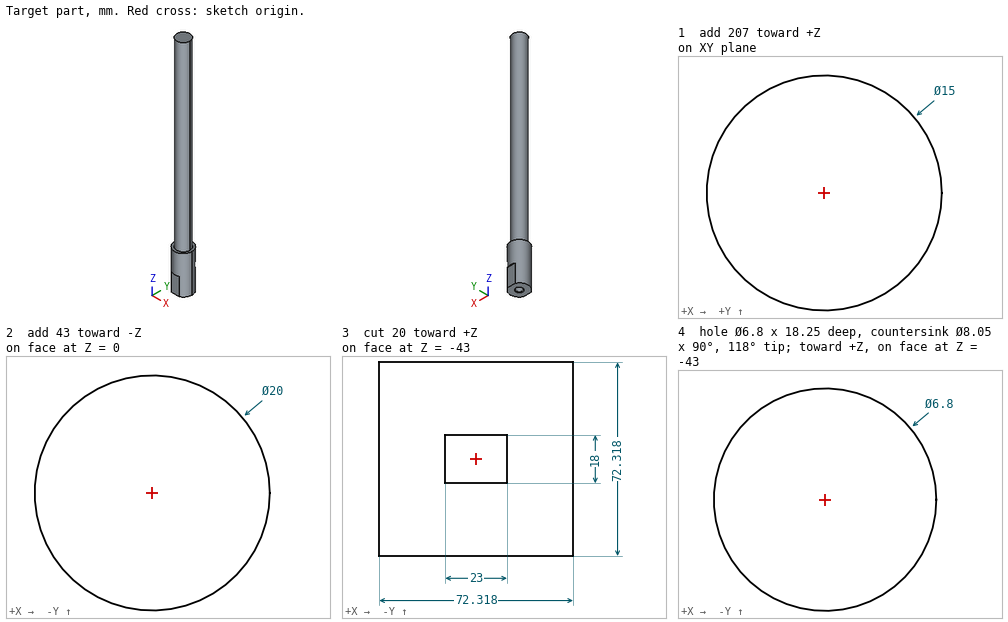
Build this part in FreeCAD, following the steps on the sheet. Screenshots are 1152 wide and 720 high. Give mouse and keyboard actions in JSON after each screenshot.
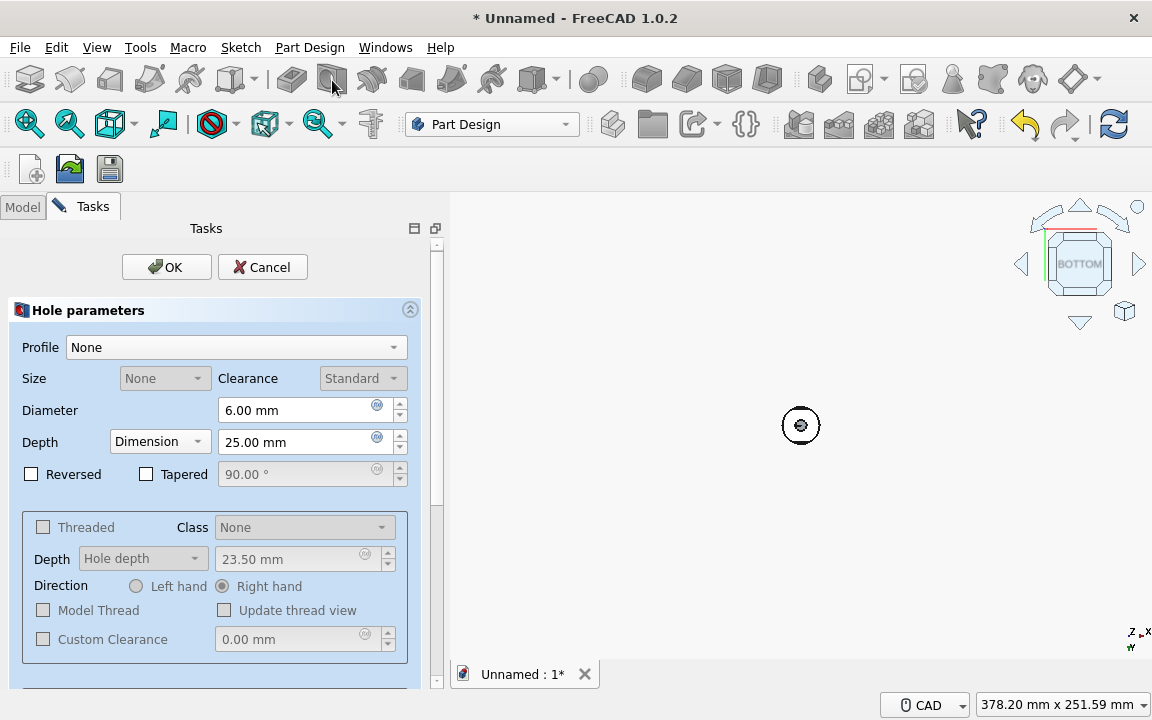
{"action": "triple_click", "coordinate": [305, 410]}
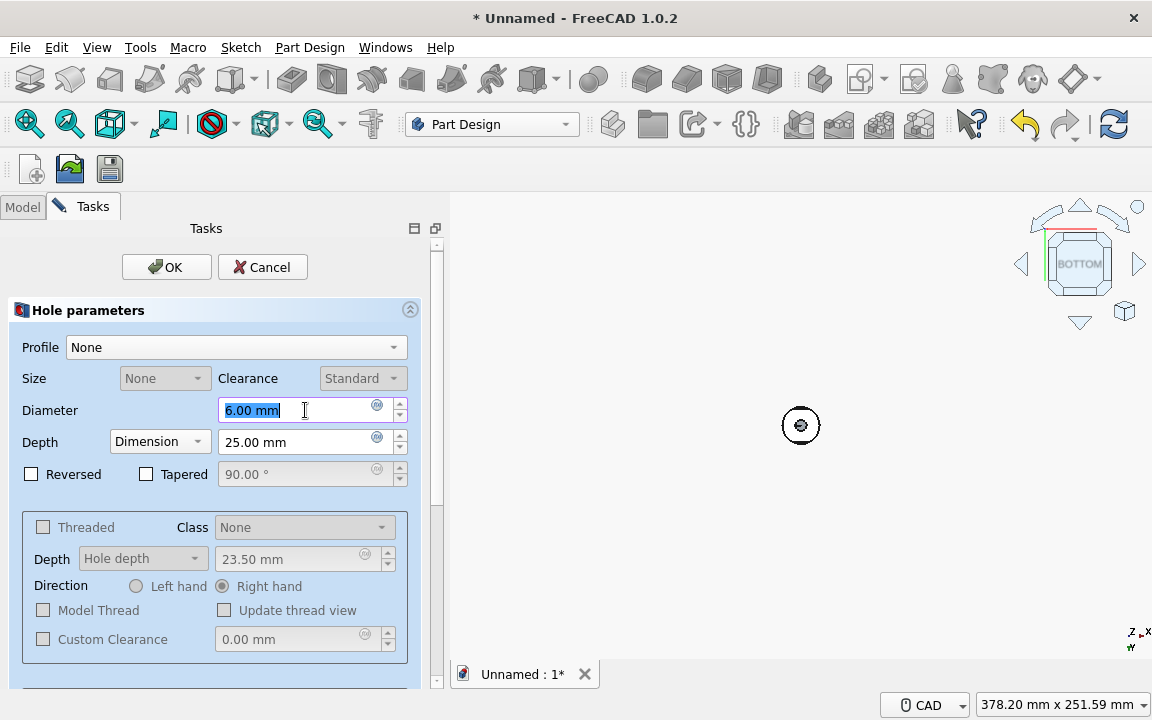
{"action": "type", "text": "6.8"}
{"action": "key", "text": "Tab"}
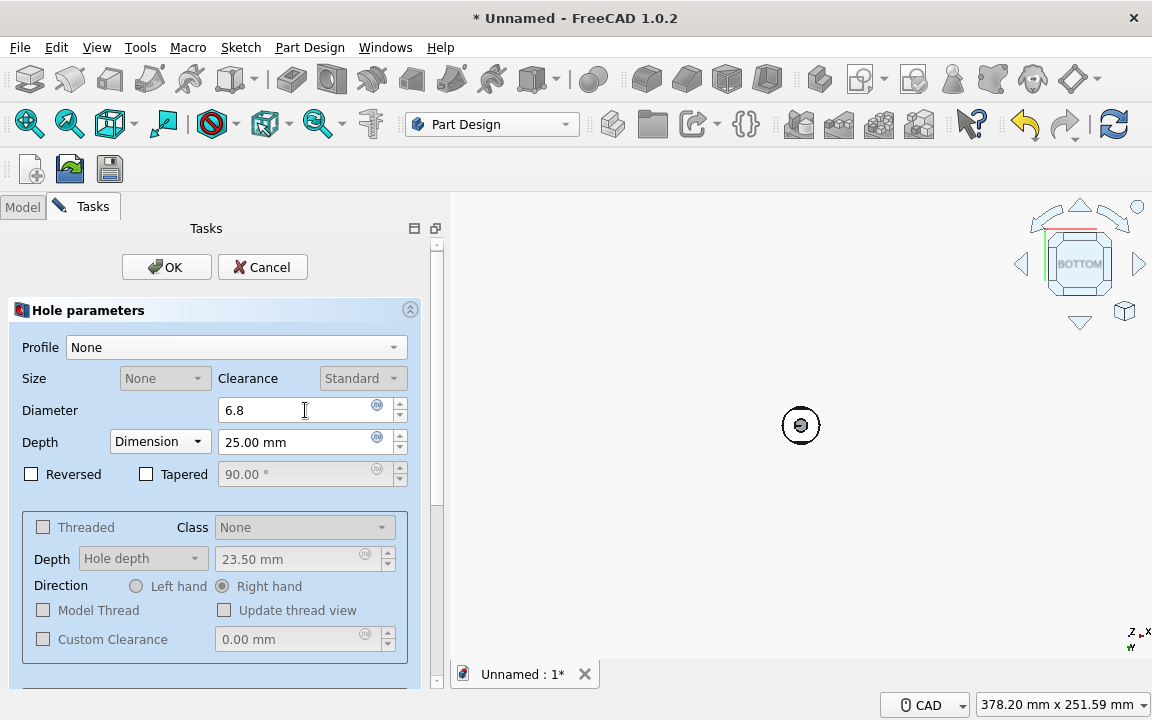
{"action": "triple_click", "coordinate": [305, 442]}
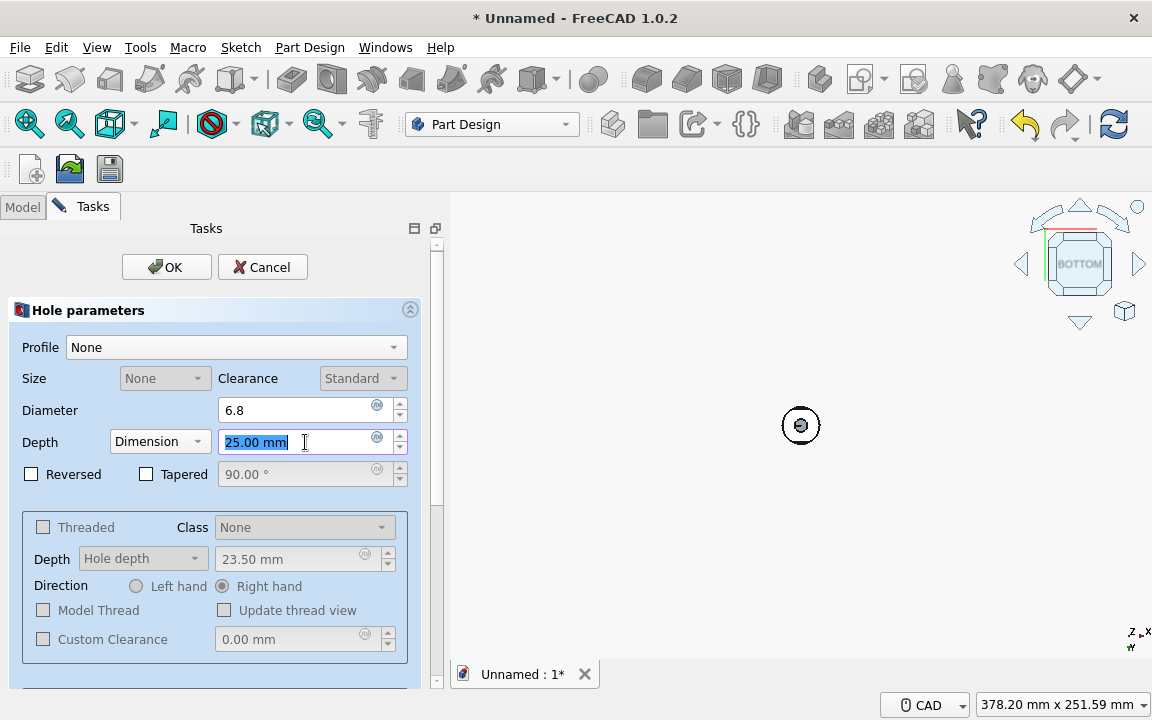
{"action": "type", "text": "18.25"}
{"action": "key", "text": "Tab"}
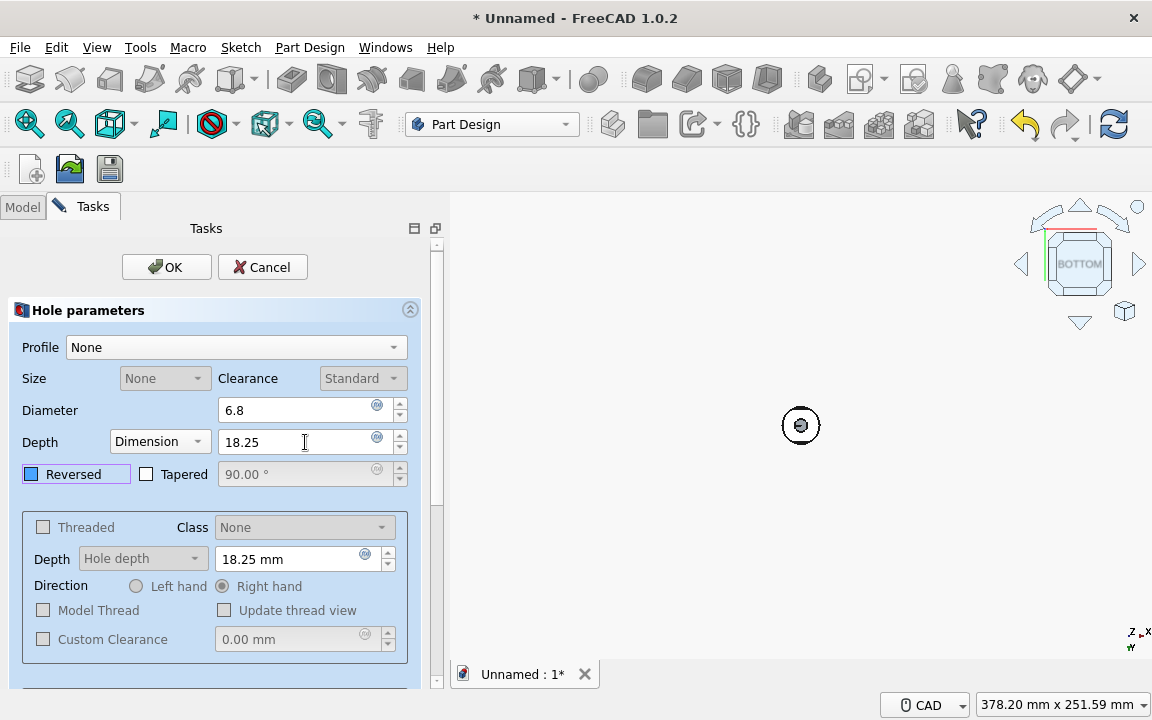
{"action": "scroll", "coordinate": [437, 463], "scroll_direction": "down", "scroll_amount": 2}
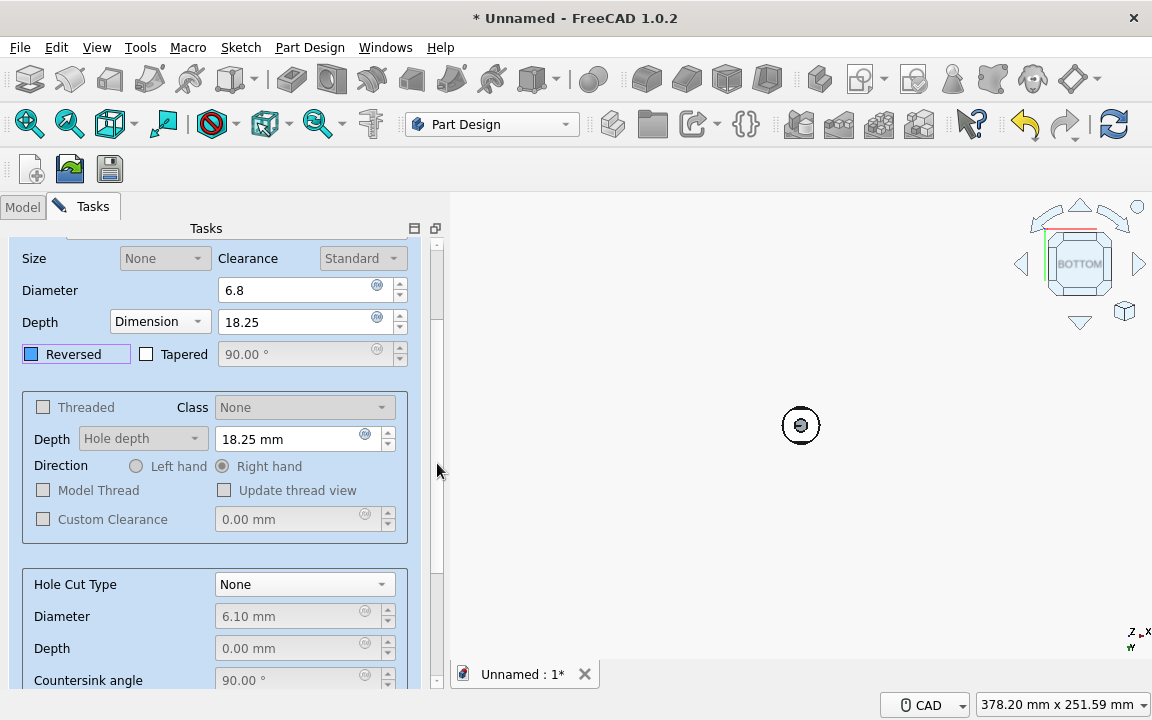
{"action": "left_click", "coordinate": [306, 584]}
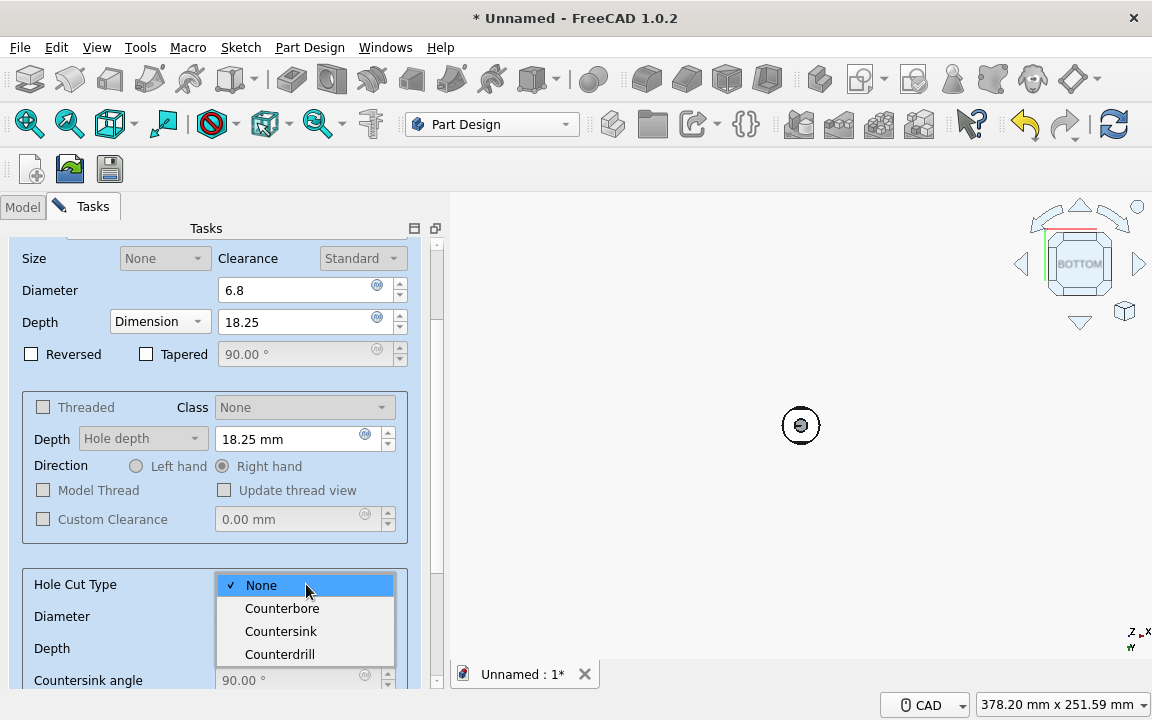
{"action": "left_click", "coordinate": [304, 632]}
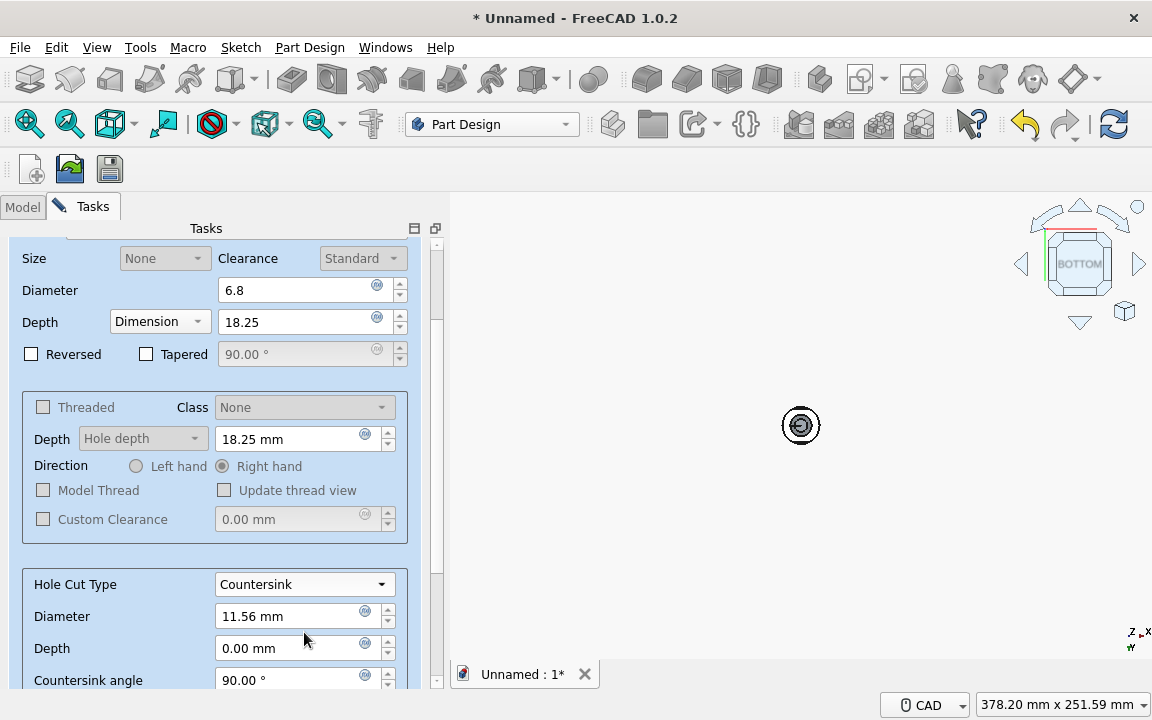
{"action": "triple_click", "coordinate": [298, 616]}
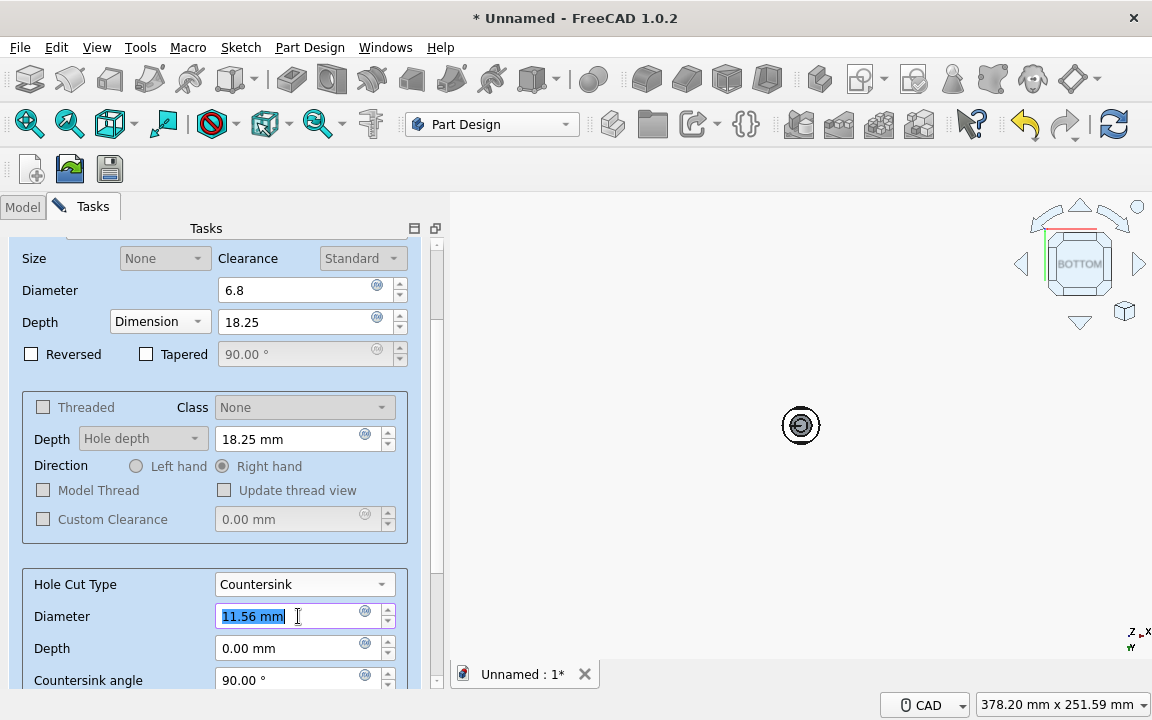
{"action": "type", "text": "8.05"}
{"action": "key", "text": "Tab"}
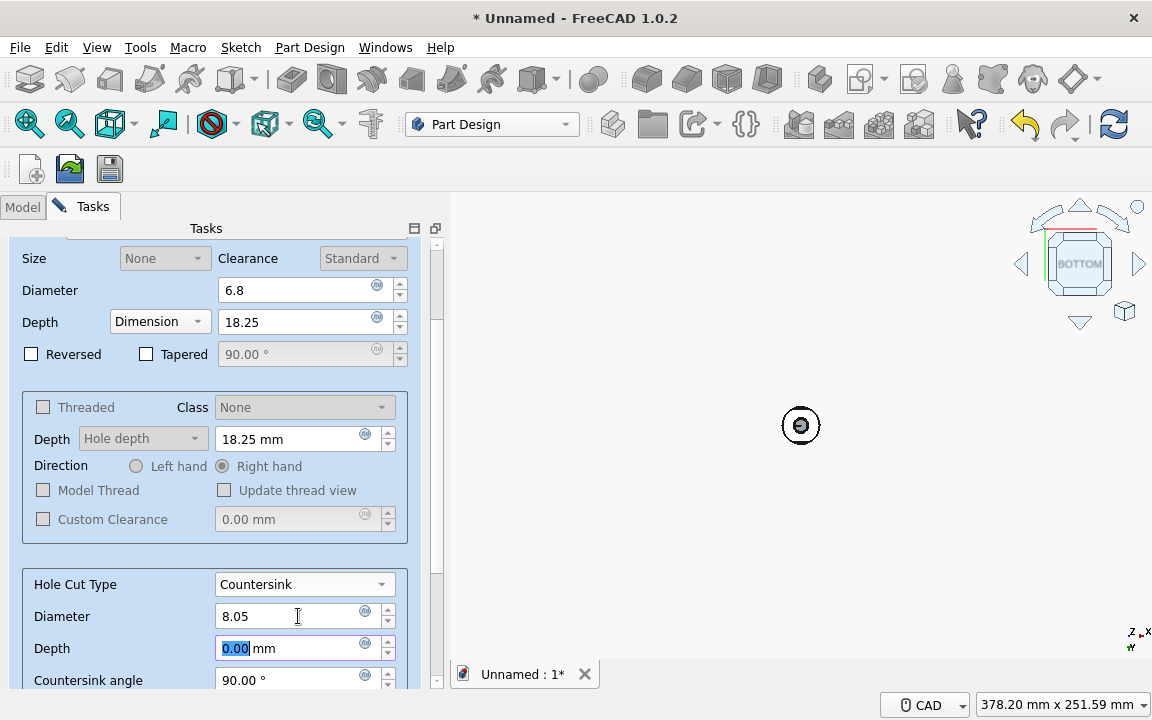
{"action": "scroll", "coordinate": [437, 463], "scroll_direction": "up", "scroll_amount": 3}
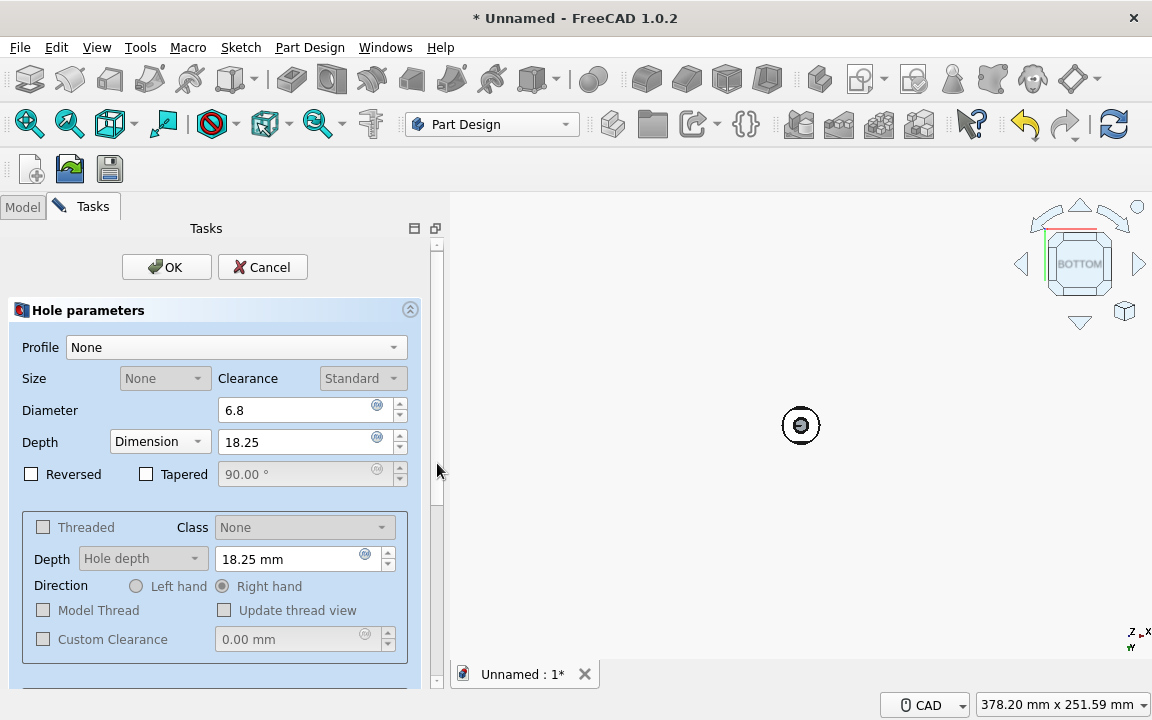
{"action": "left_click", "coordinate": [167, 267]}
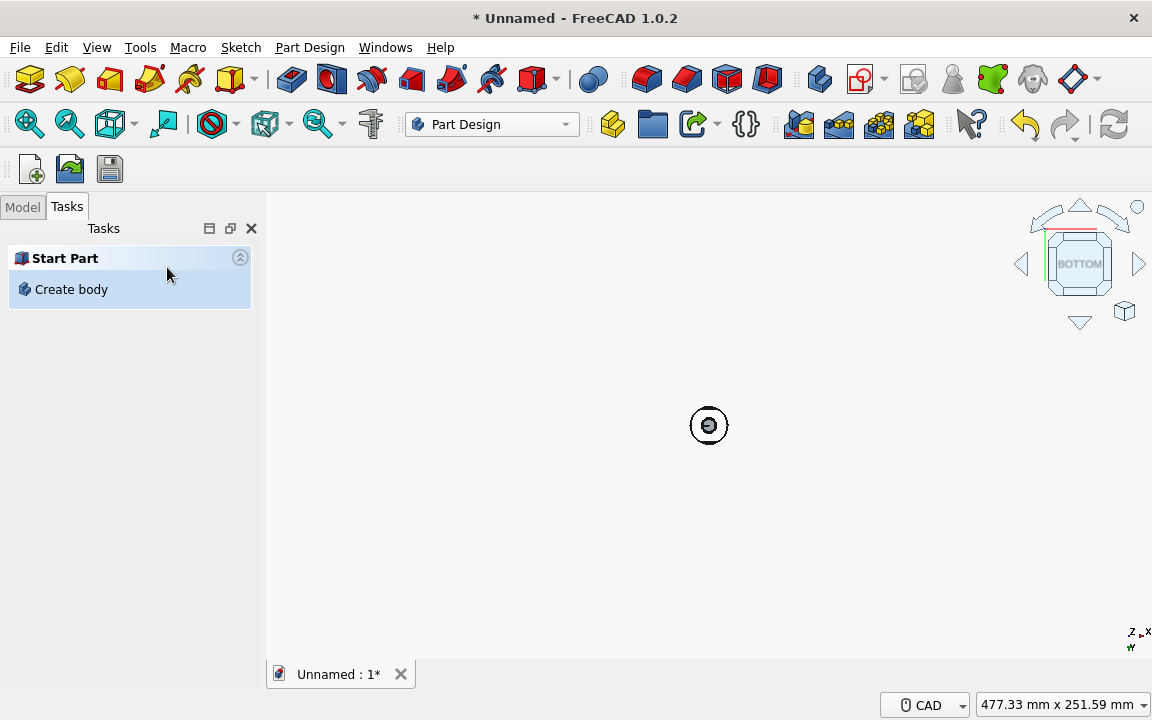
{"action": "key", "text": "0"}